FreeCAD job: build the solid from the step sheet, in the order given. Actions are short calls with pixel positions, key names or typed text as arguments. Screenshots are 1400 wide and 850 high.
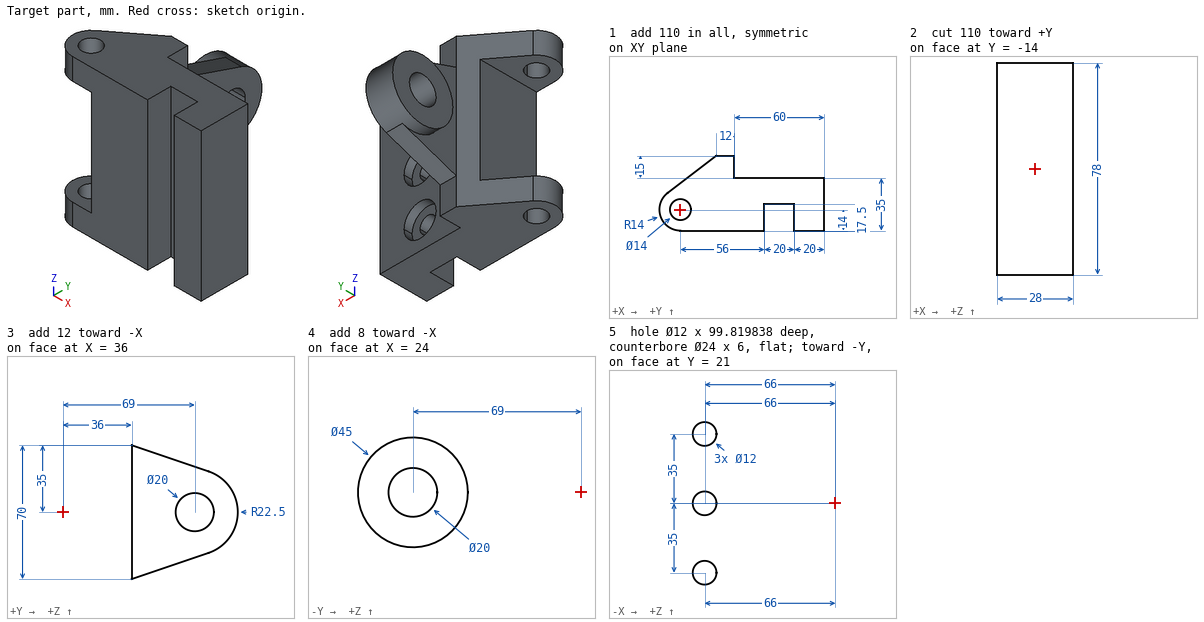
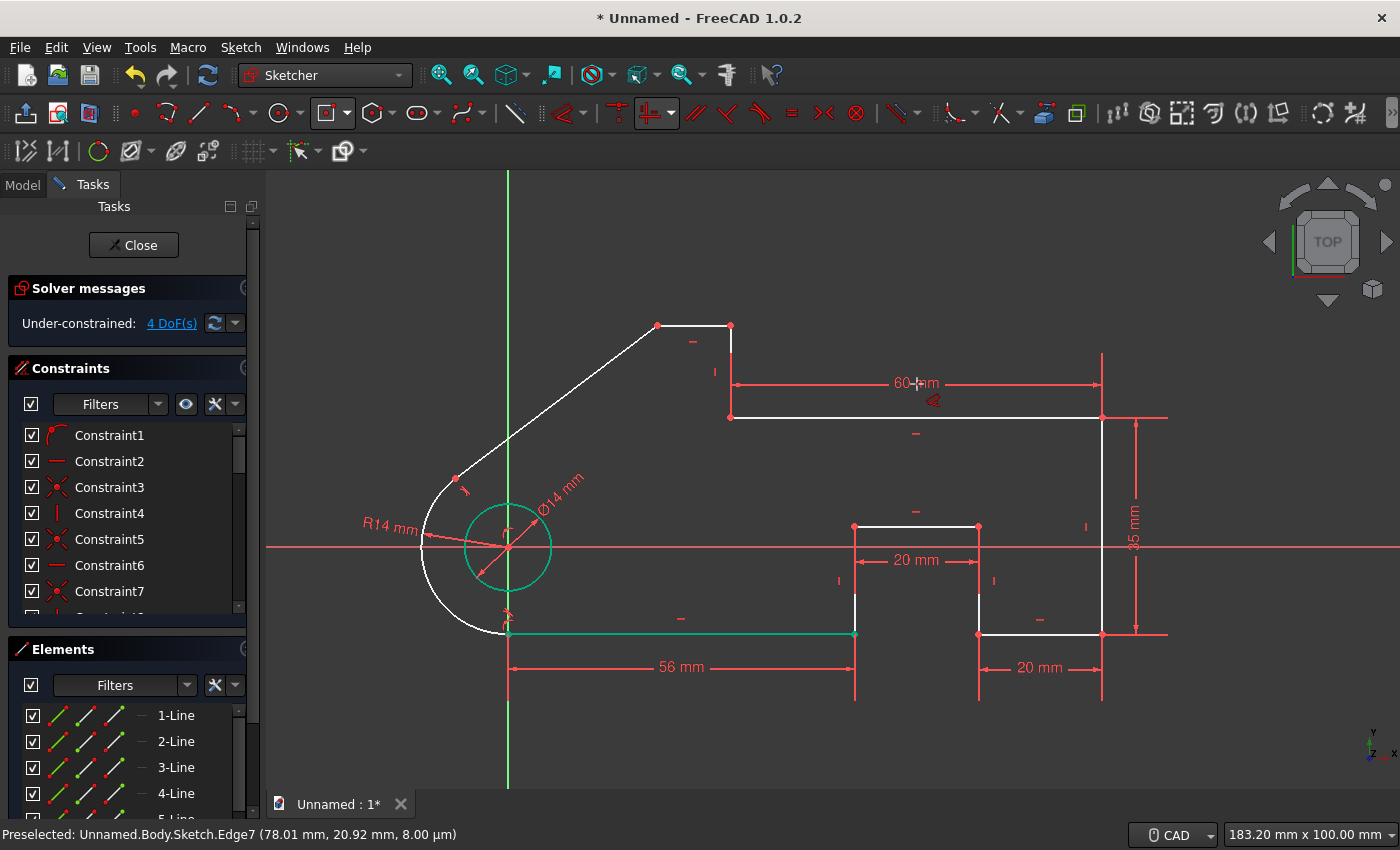
click(731, 390)
click(697, 372)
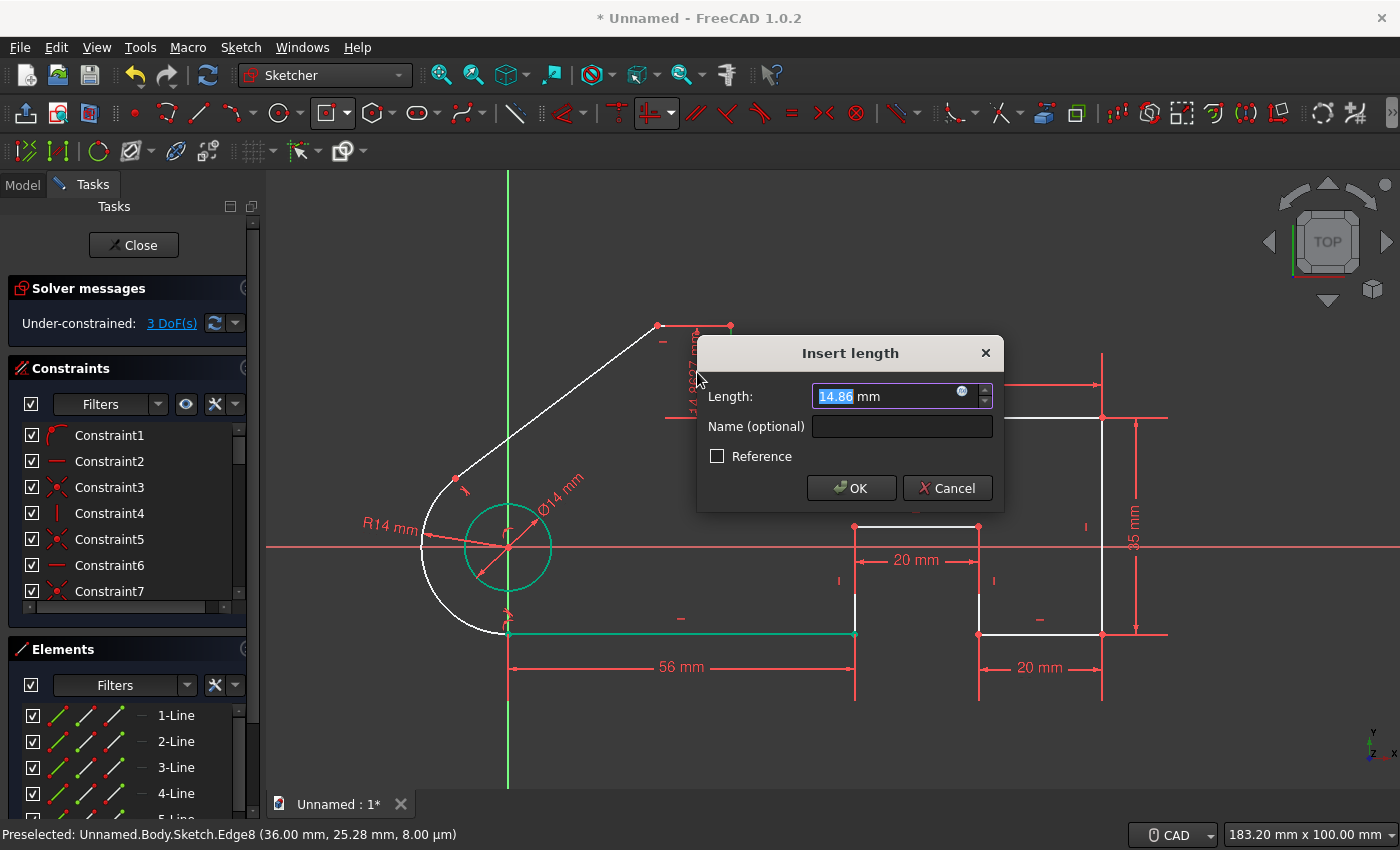
text(15)
key(Return)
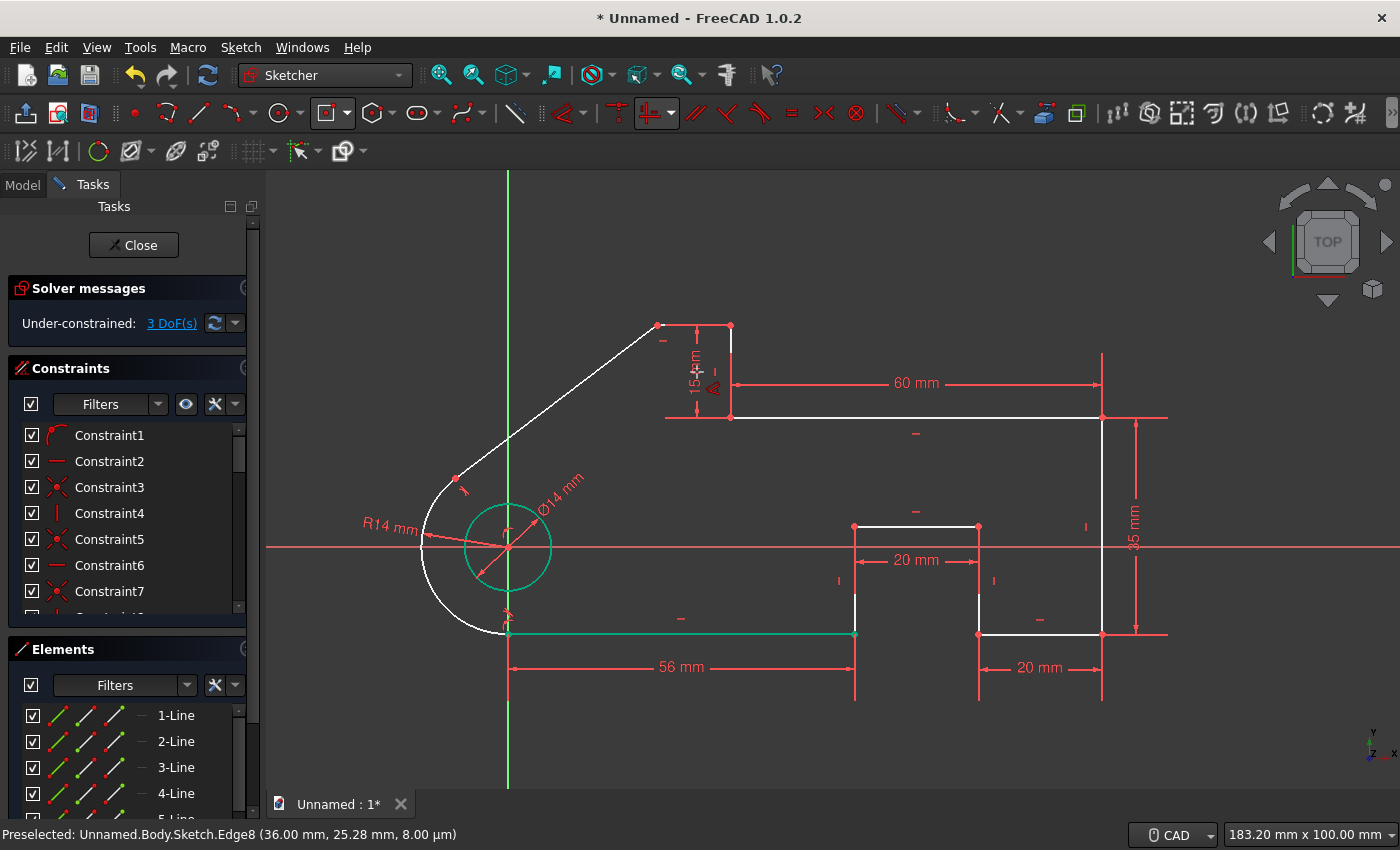
click(709, 325)
click(694, 291)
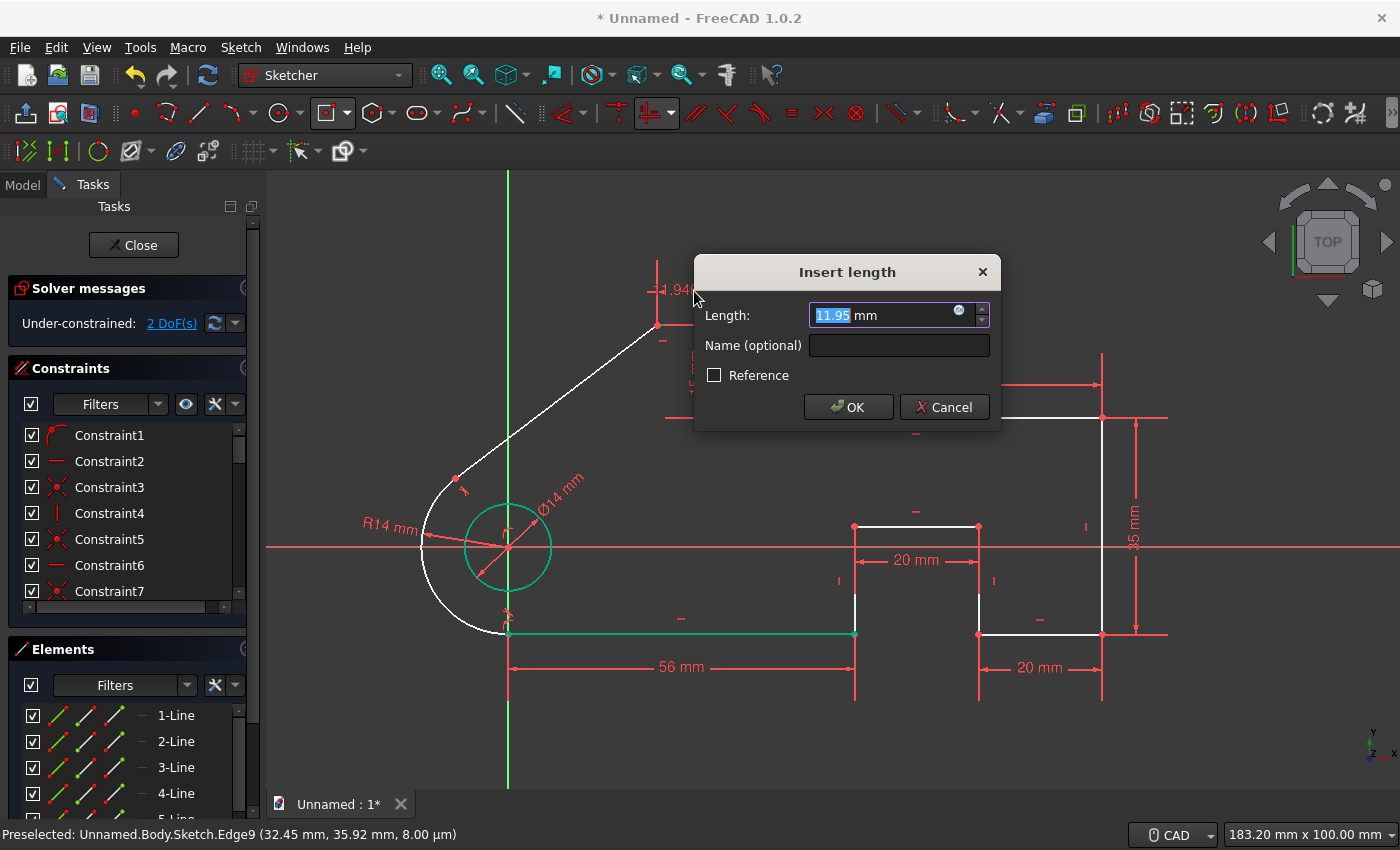
text(12)
key(Return)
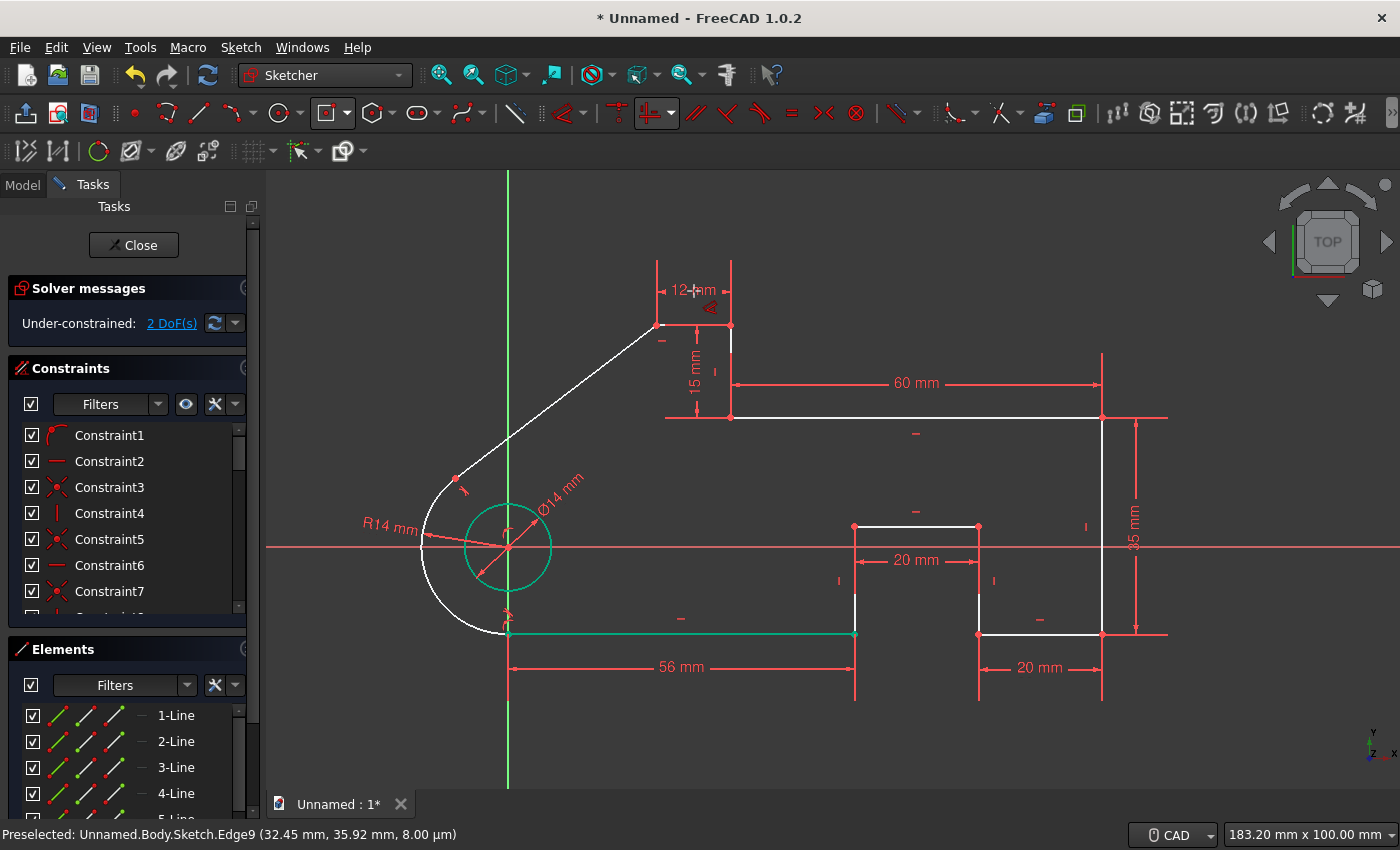
click(979, 635)
click(474, 611)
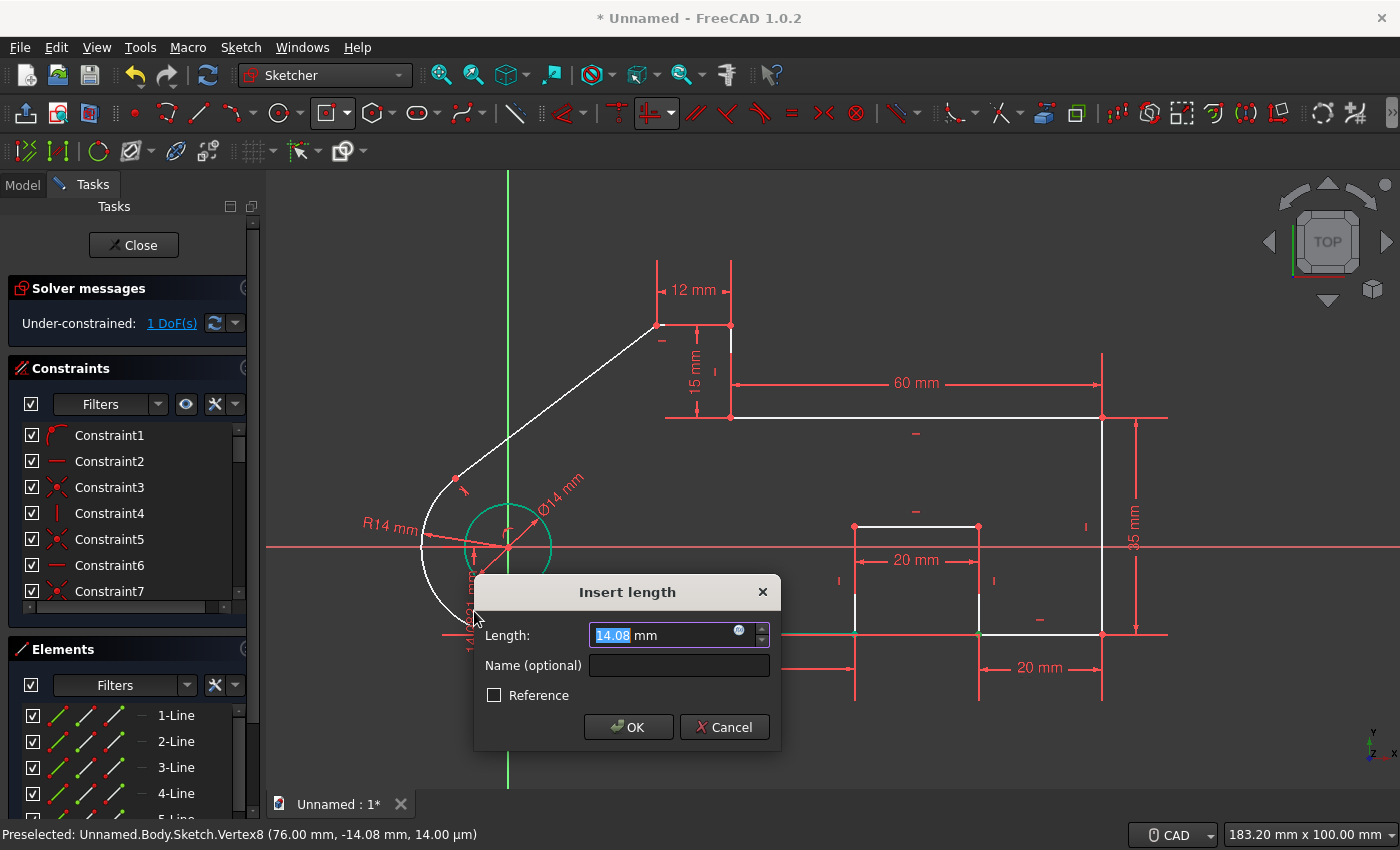
text(14)
key(Return)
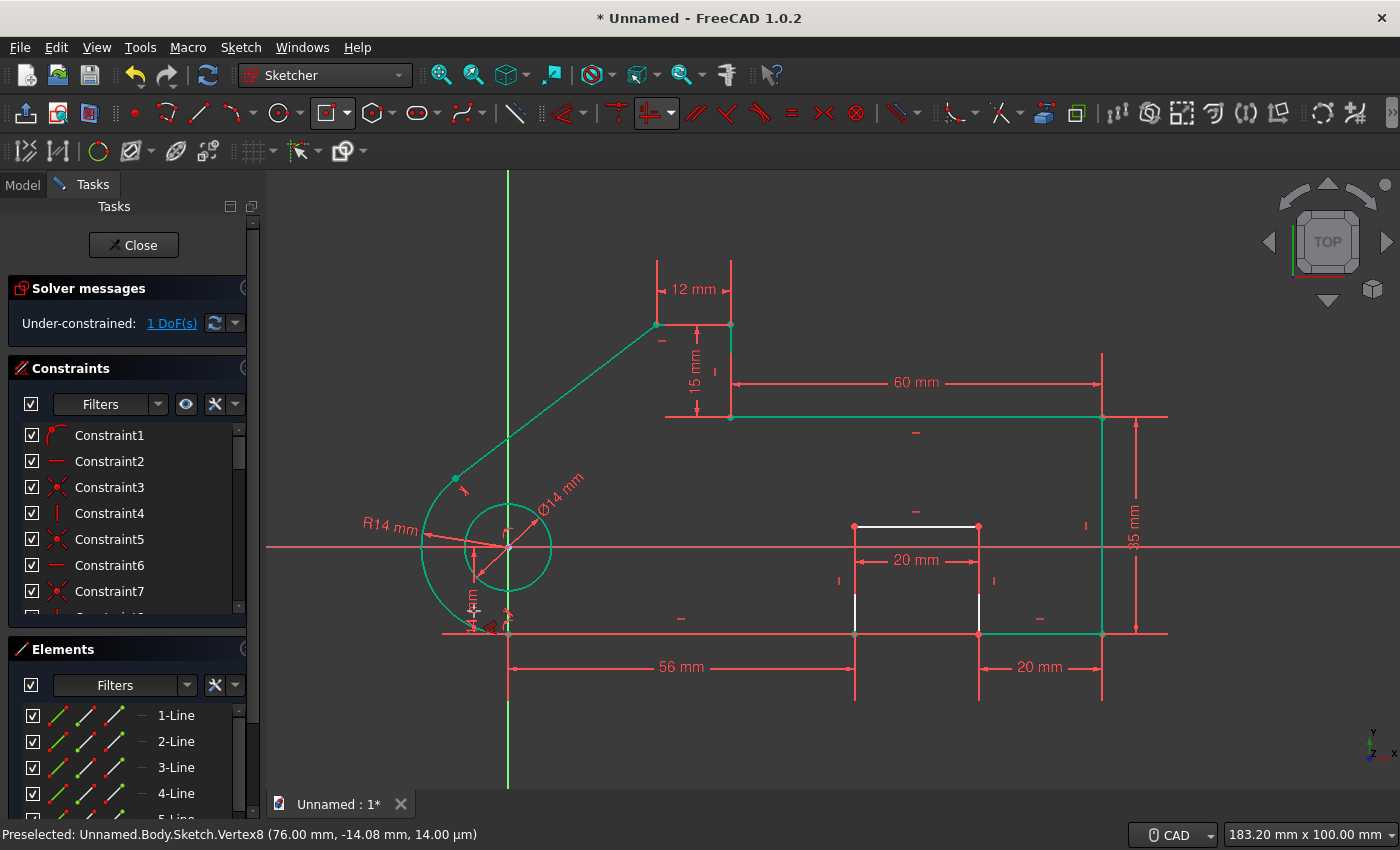
click(855, 602)
click(889, 605)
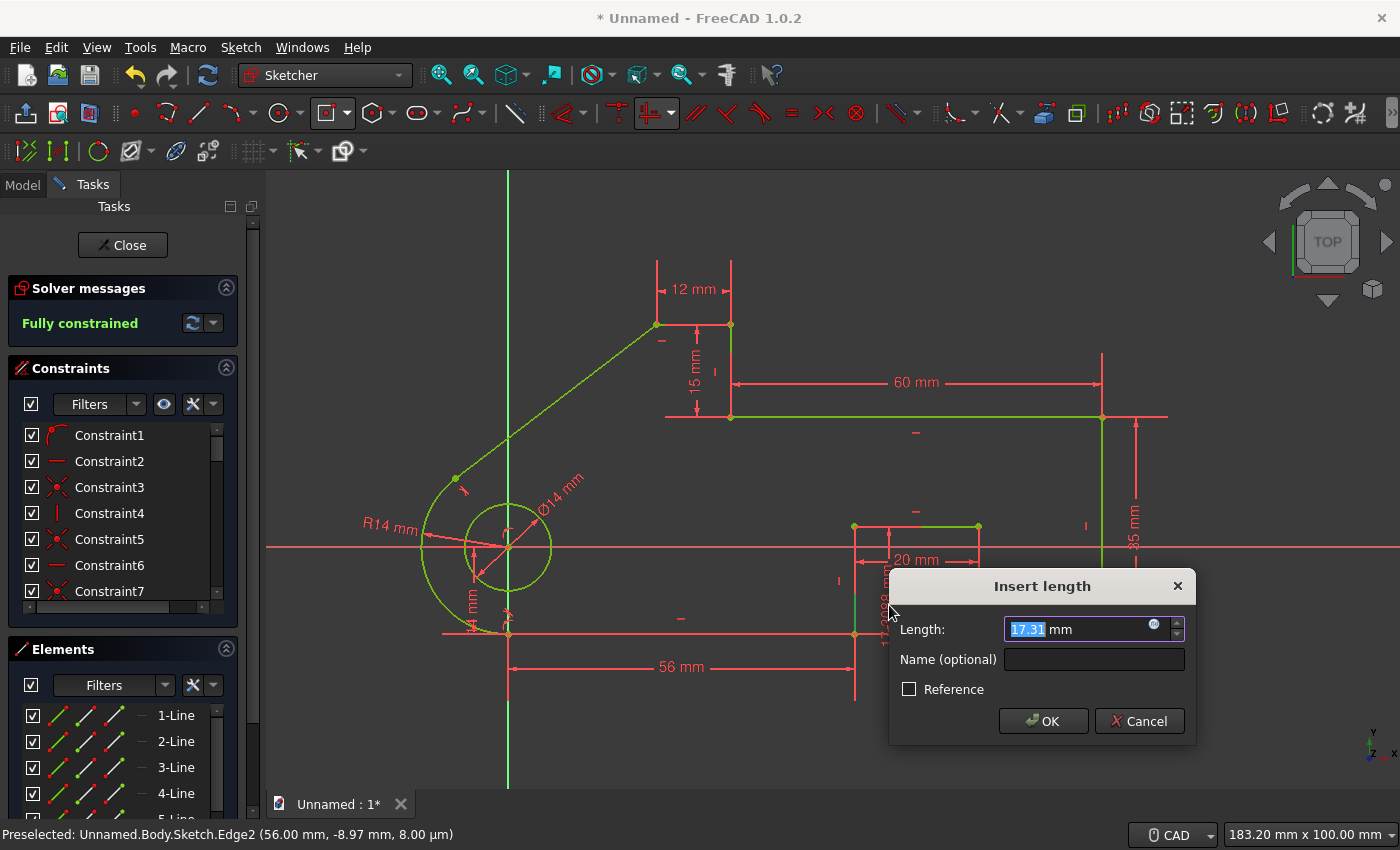
text(17.5)
key(Return)
key(Escape)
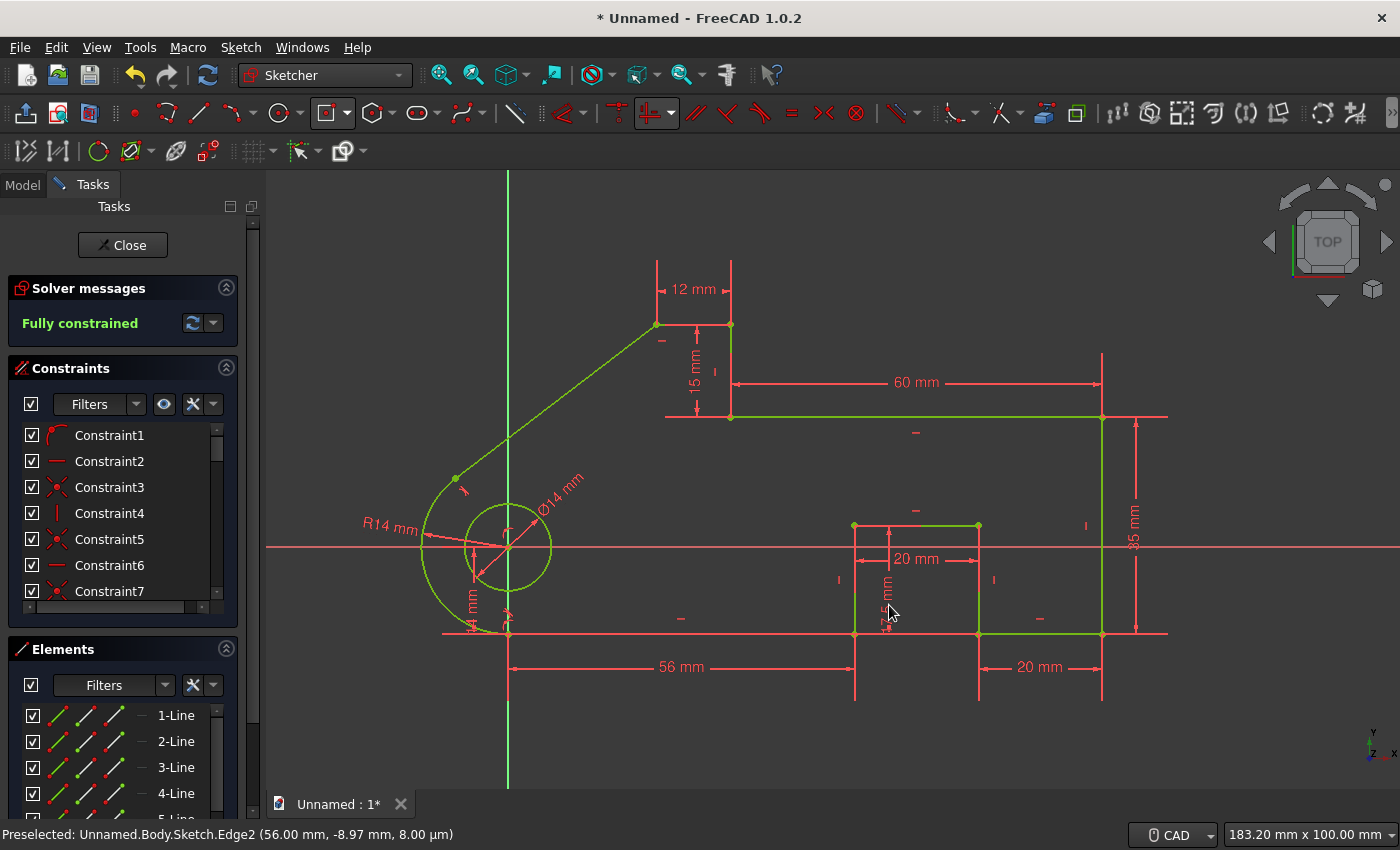
click(123, 245)